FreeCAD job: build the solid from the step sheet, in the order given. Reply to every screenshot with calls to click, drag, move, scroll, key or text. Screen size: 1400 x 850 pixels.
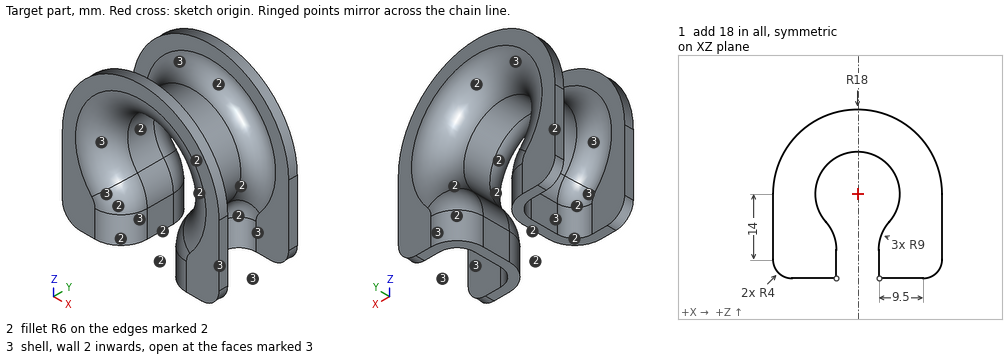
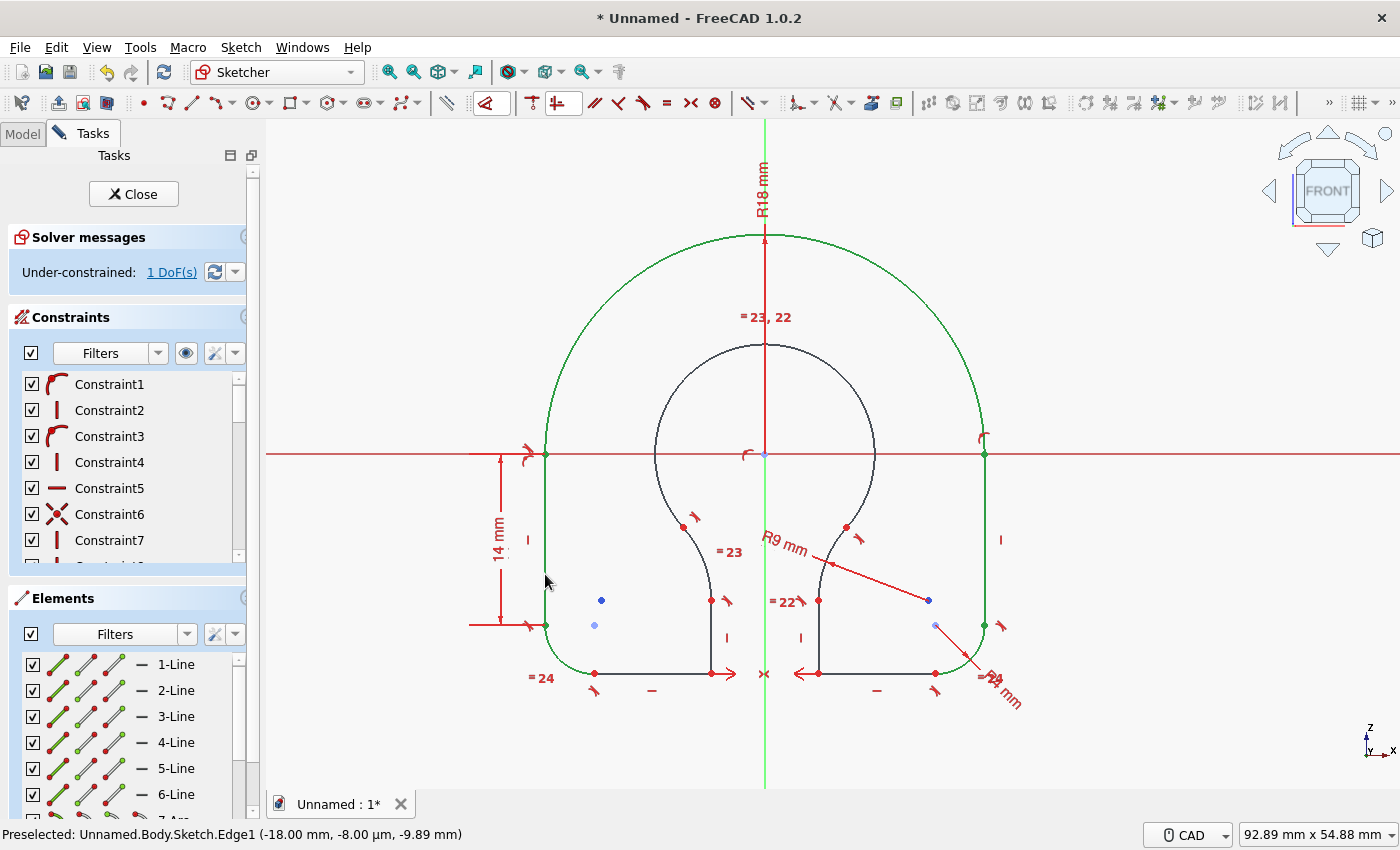
click(901, 674)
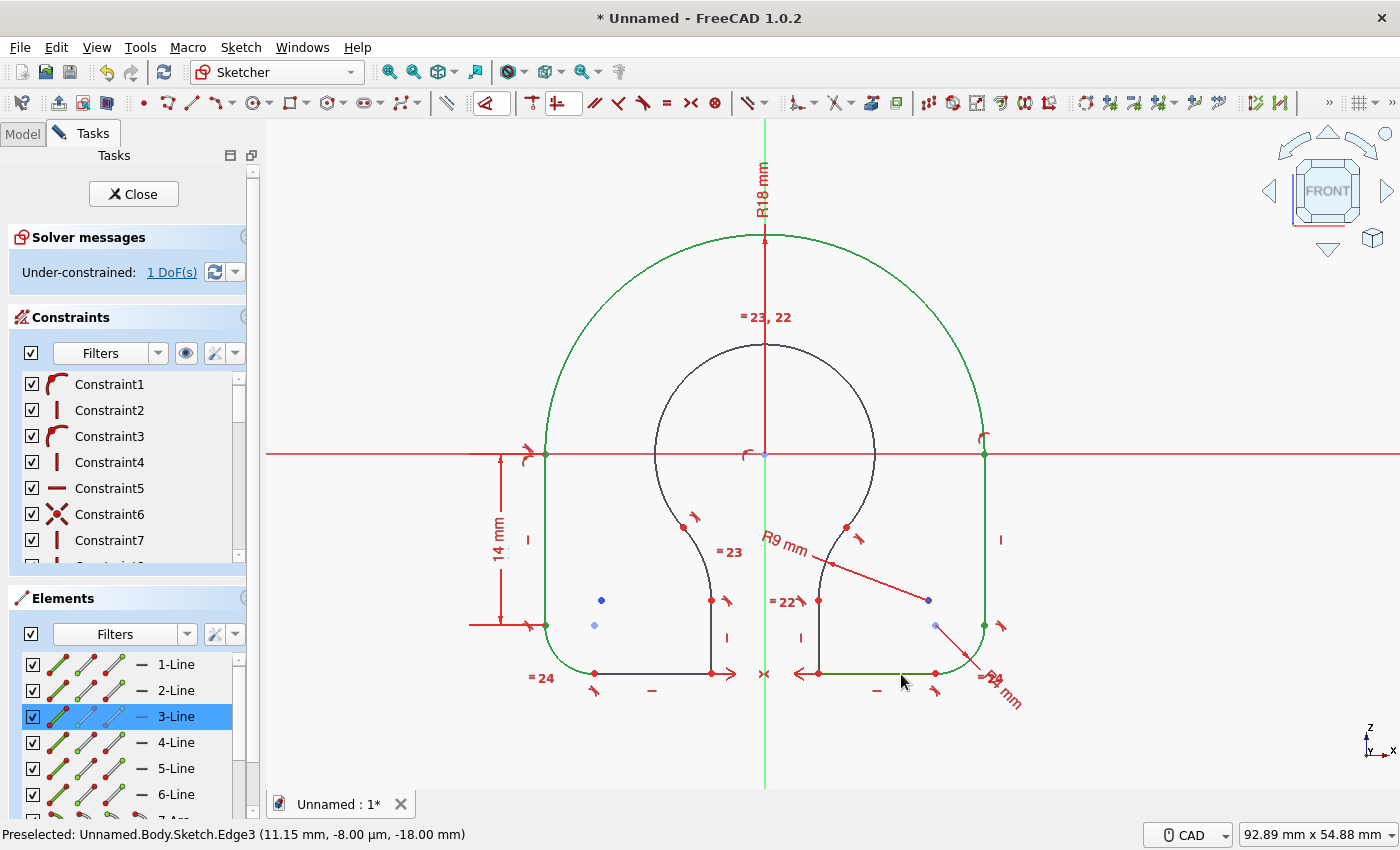
key(l)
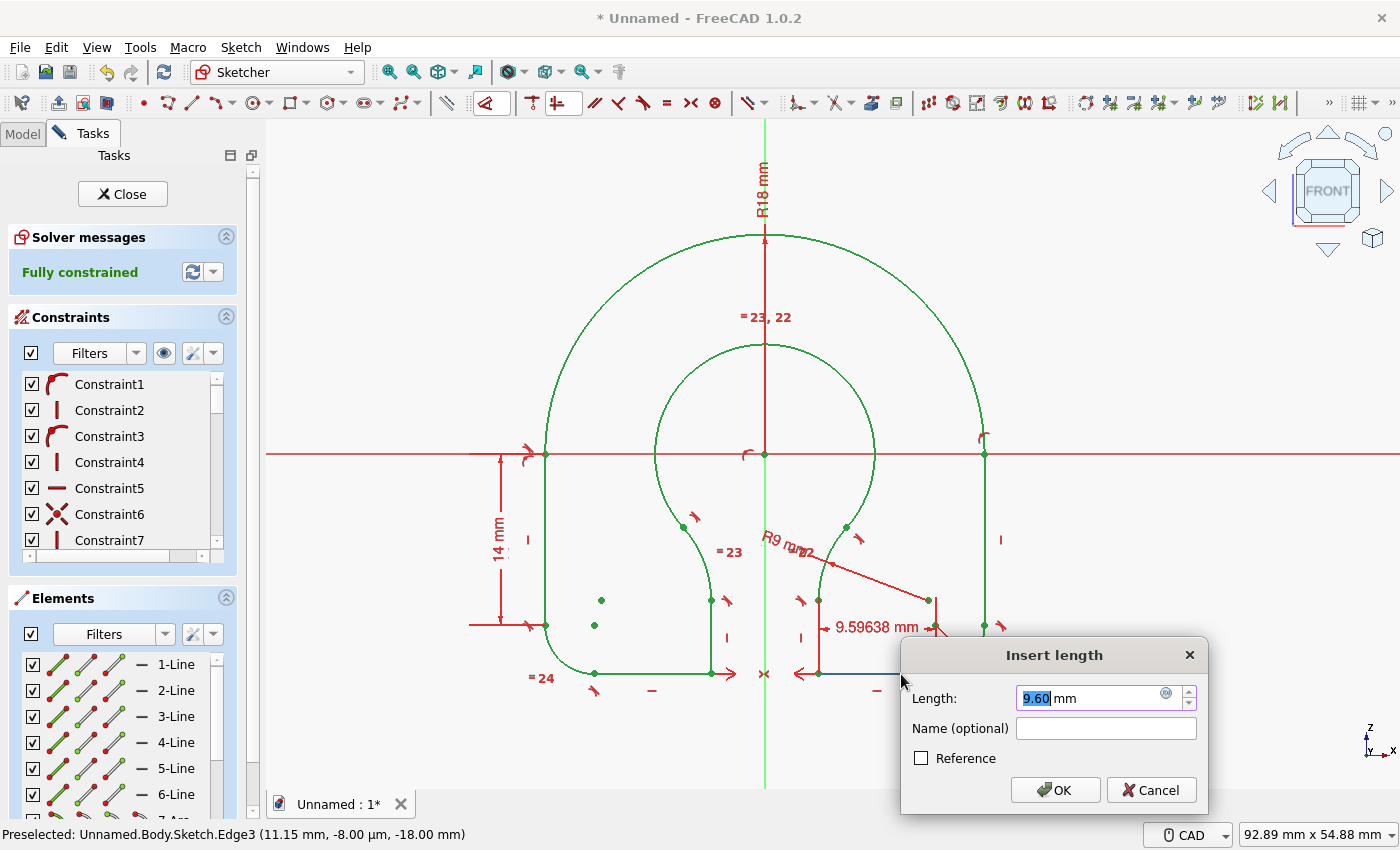
text(9.5)
key(Return)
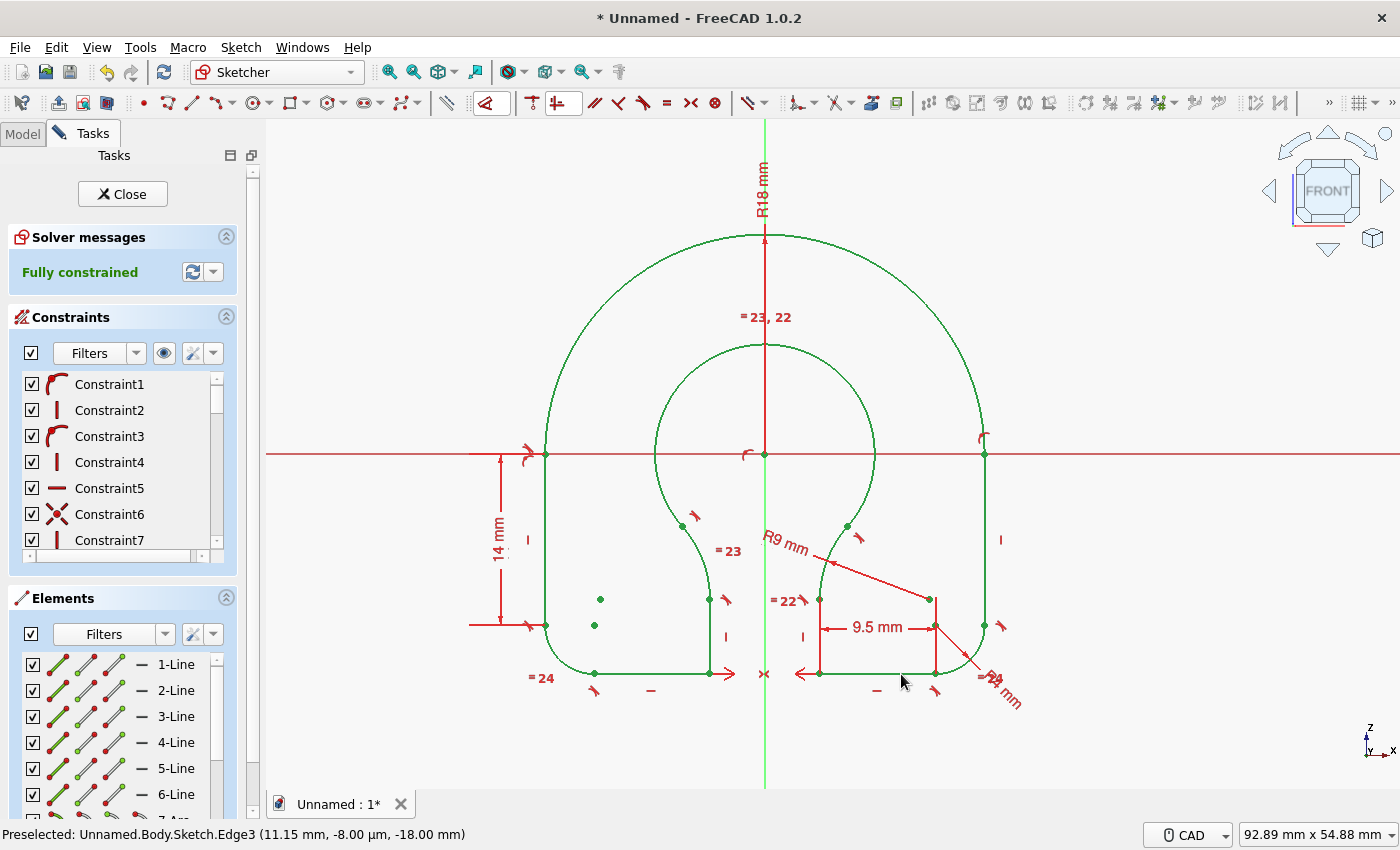
click(123, 194)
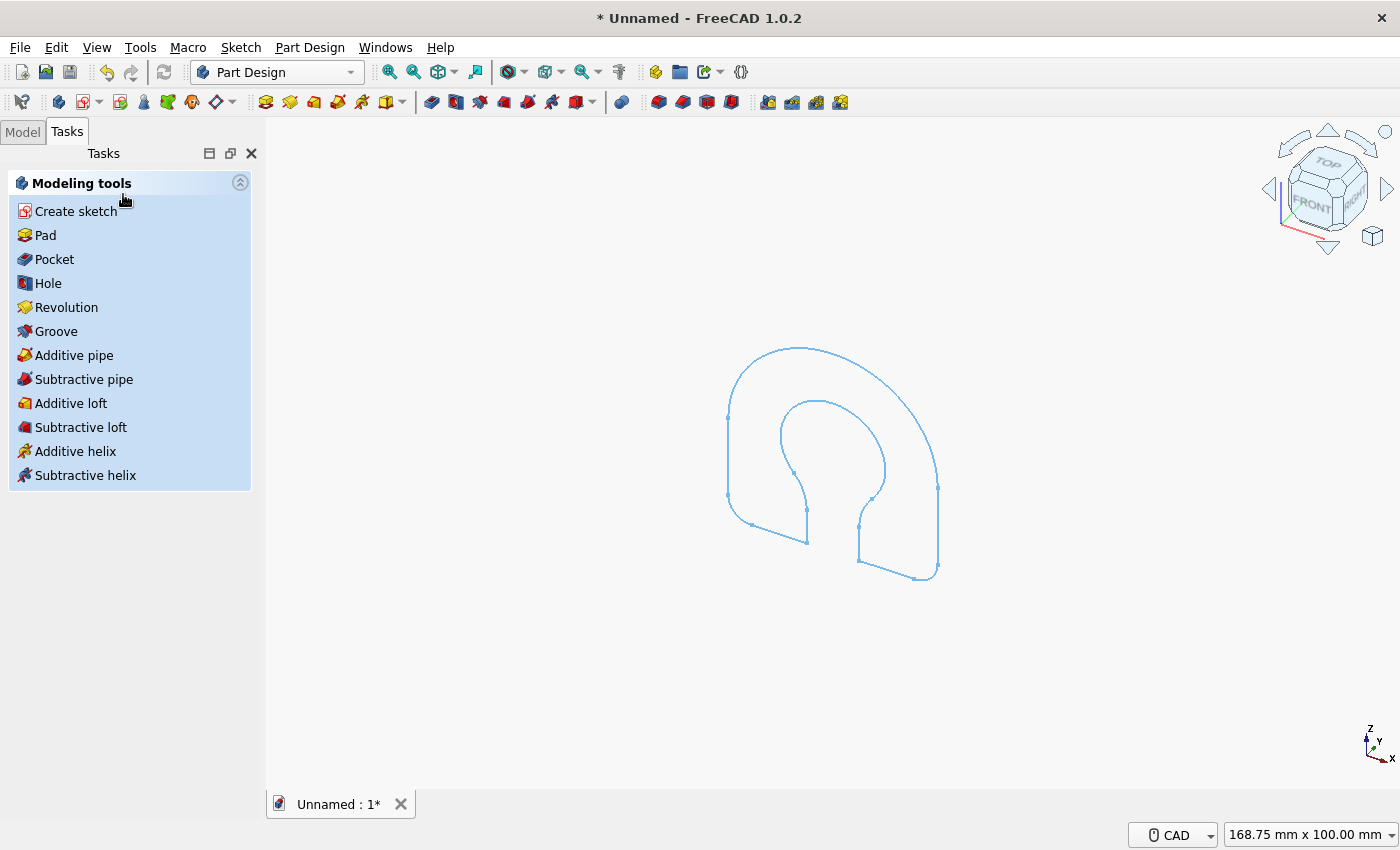
click(266, 102)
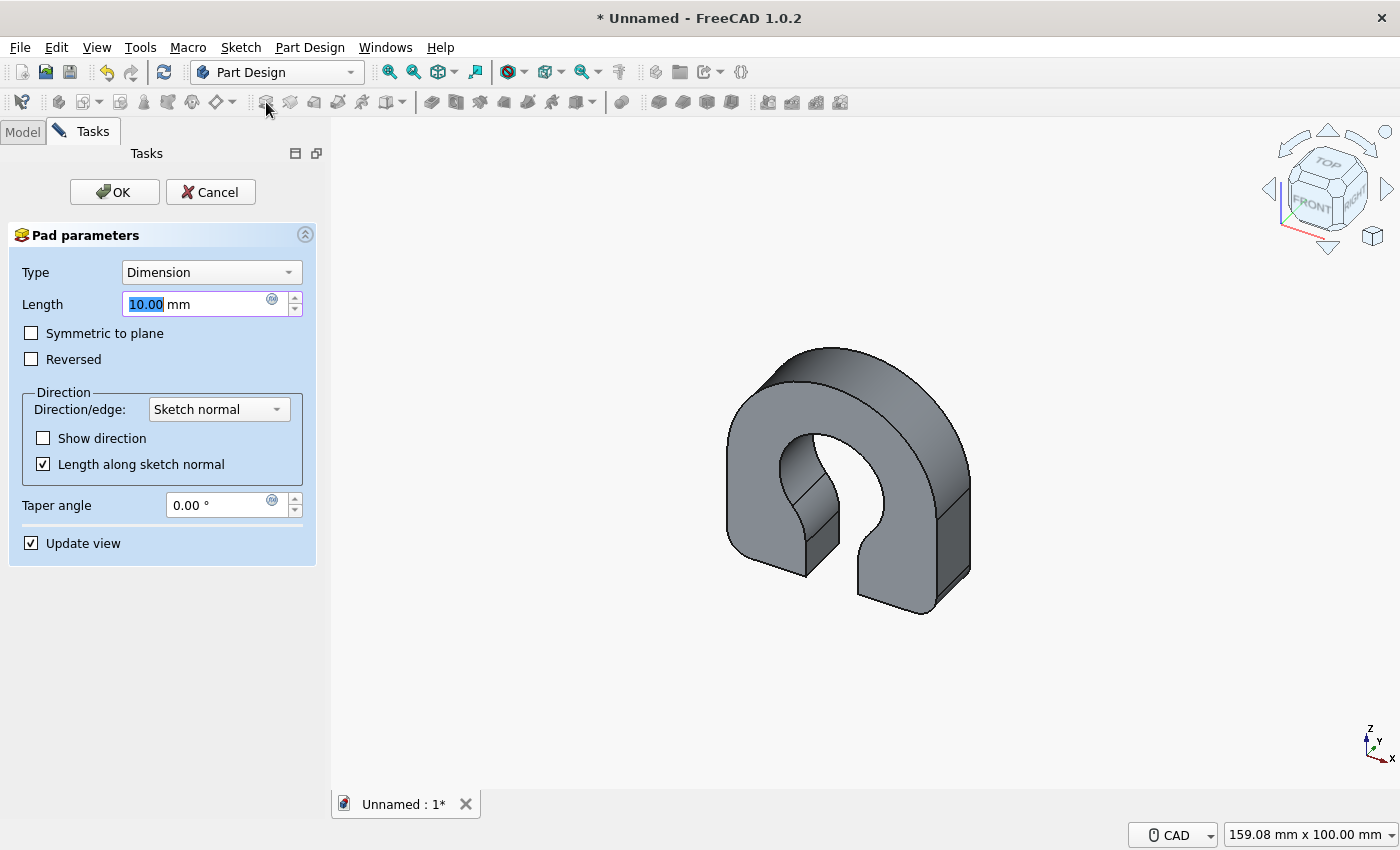
text(18)
key(Tab)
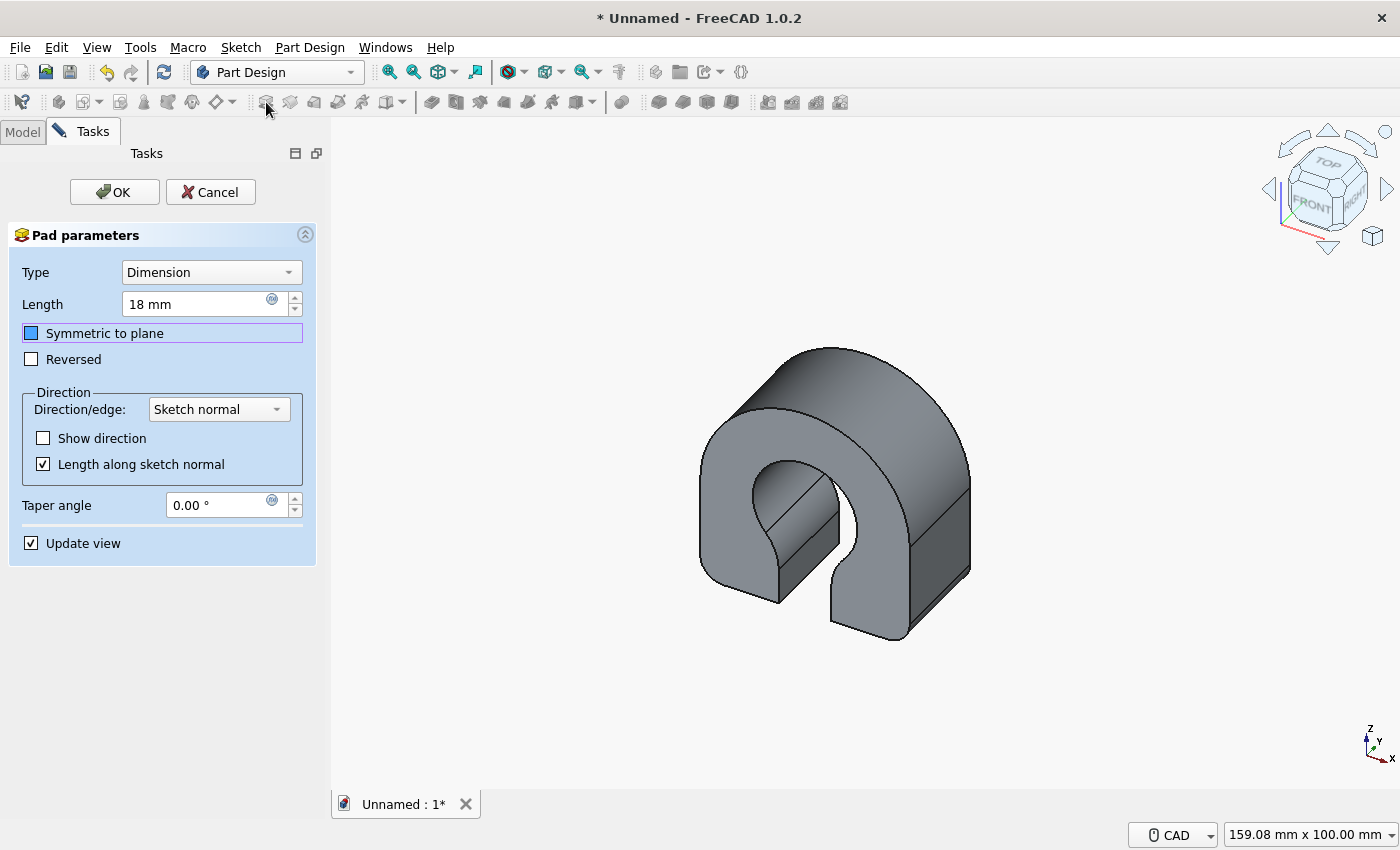
click(30, 333)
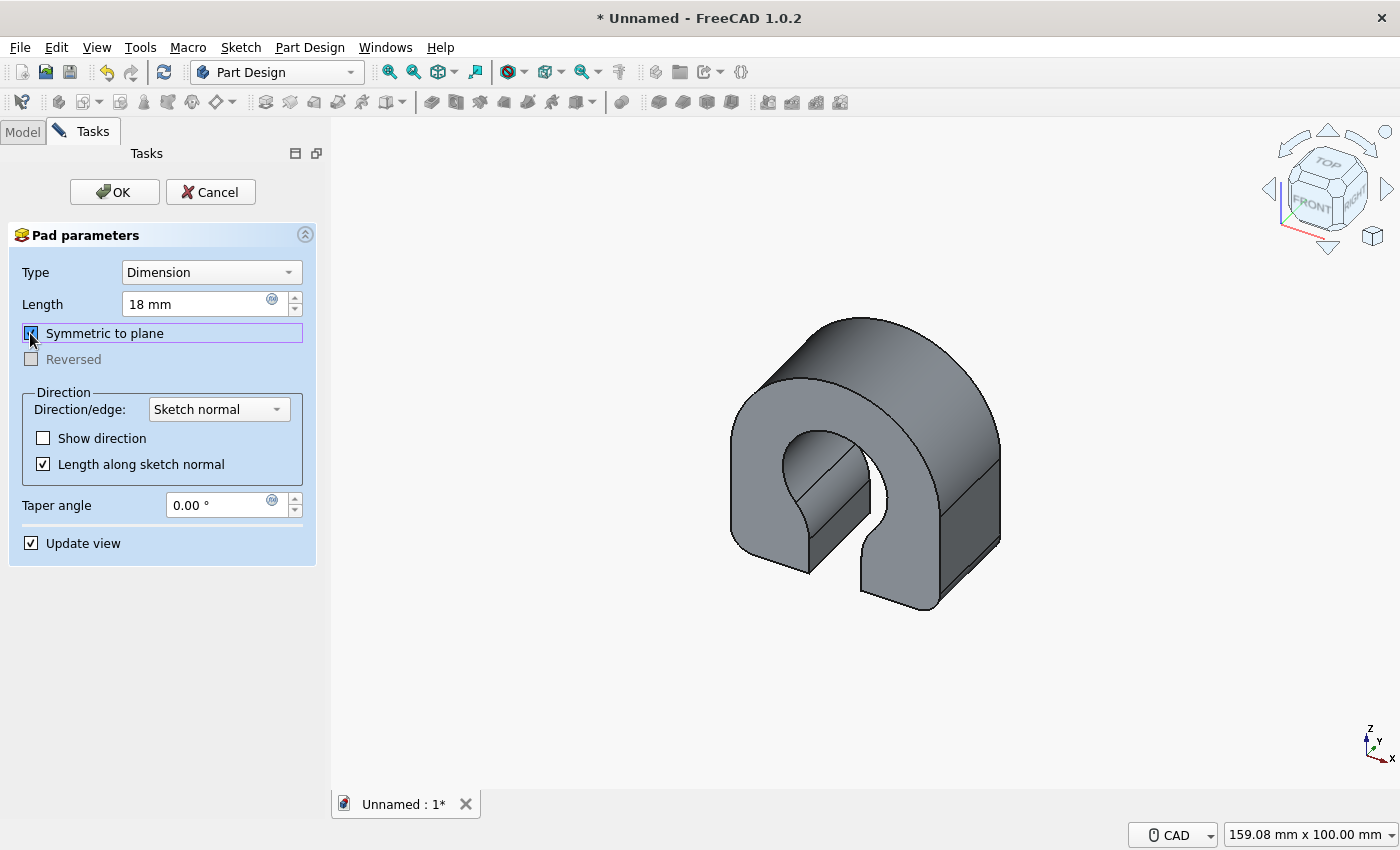
click(115, 192)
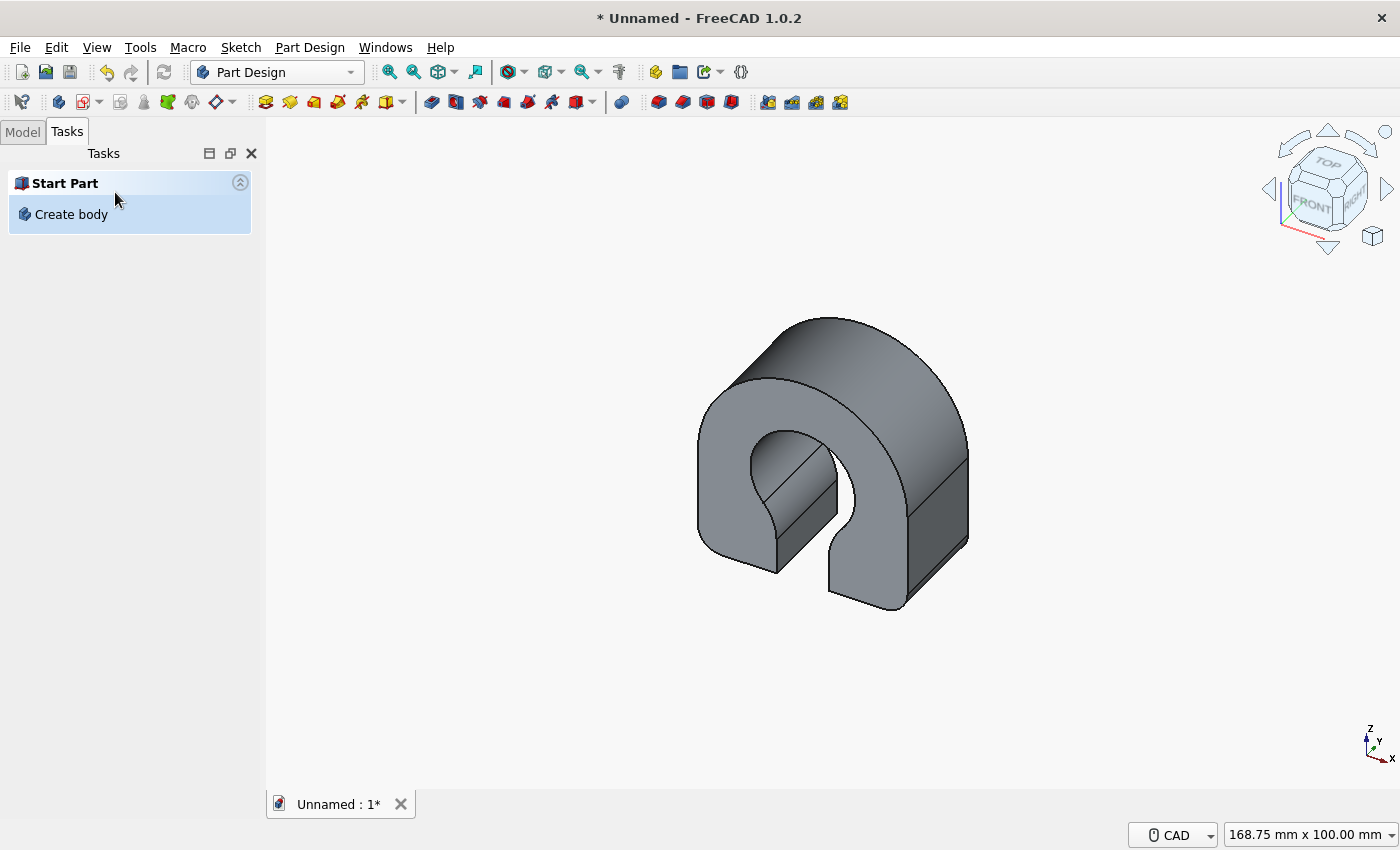
click(780, 430)